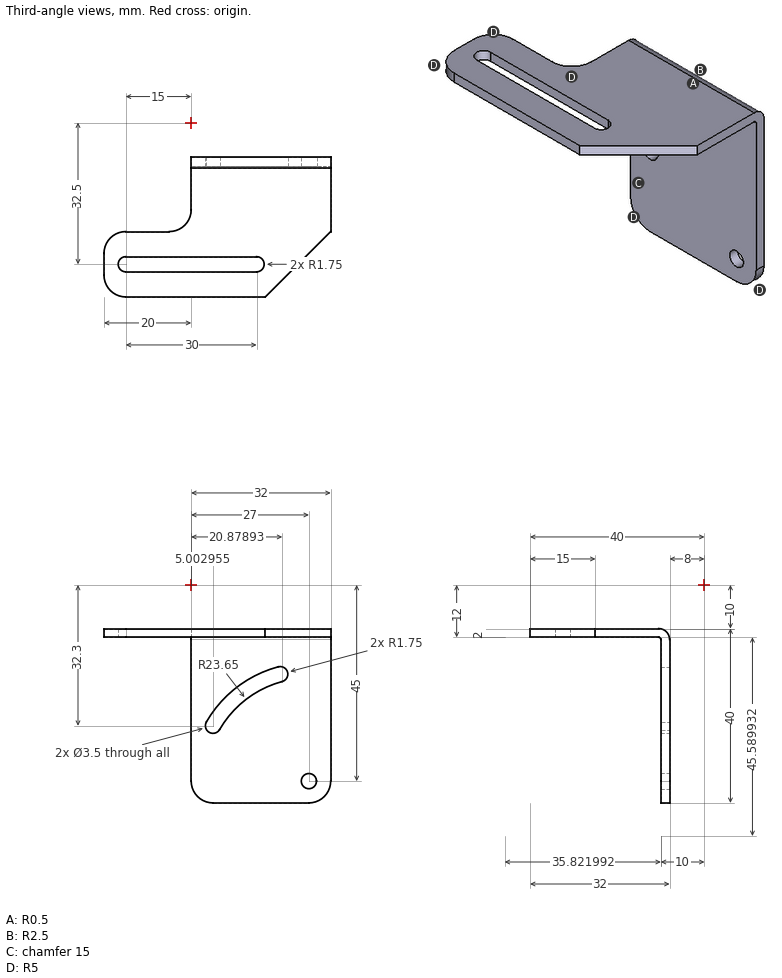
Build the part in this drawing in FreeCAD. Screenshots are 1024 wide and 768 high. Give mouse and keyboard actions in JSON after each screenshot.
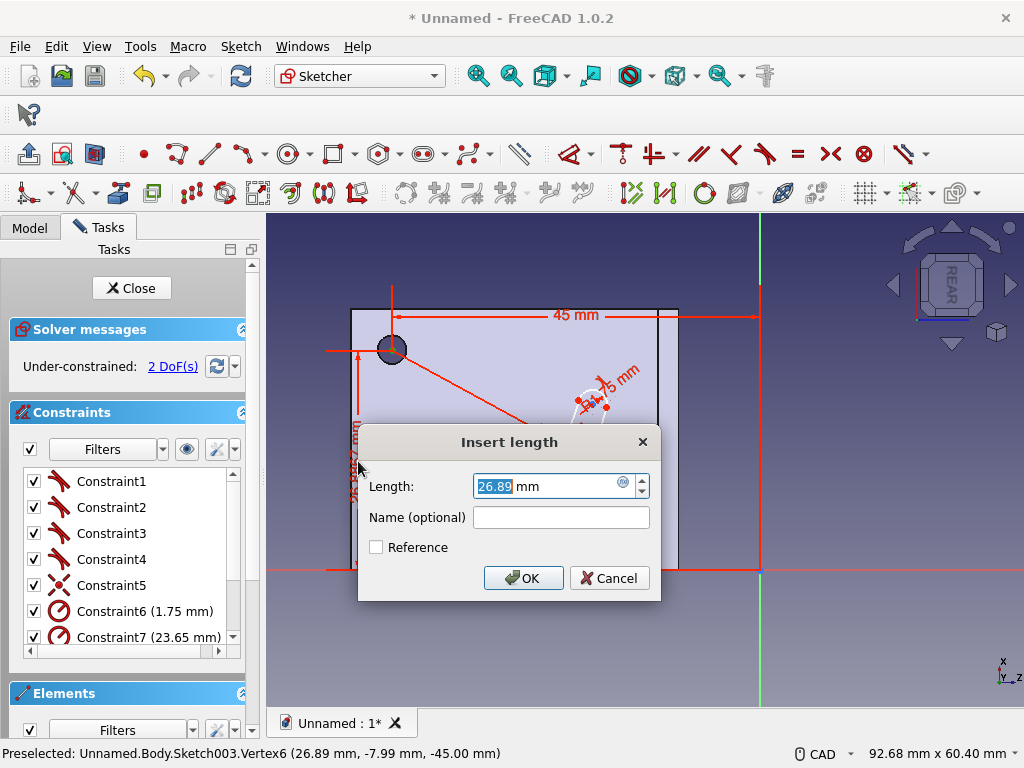
{"action": "type", "text": "27"}
{"action": "key", "text": "Return"}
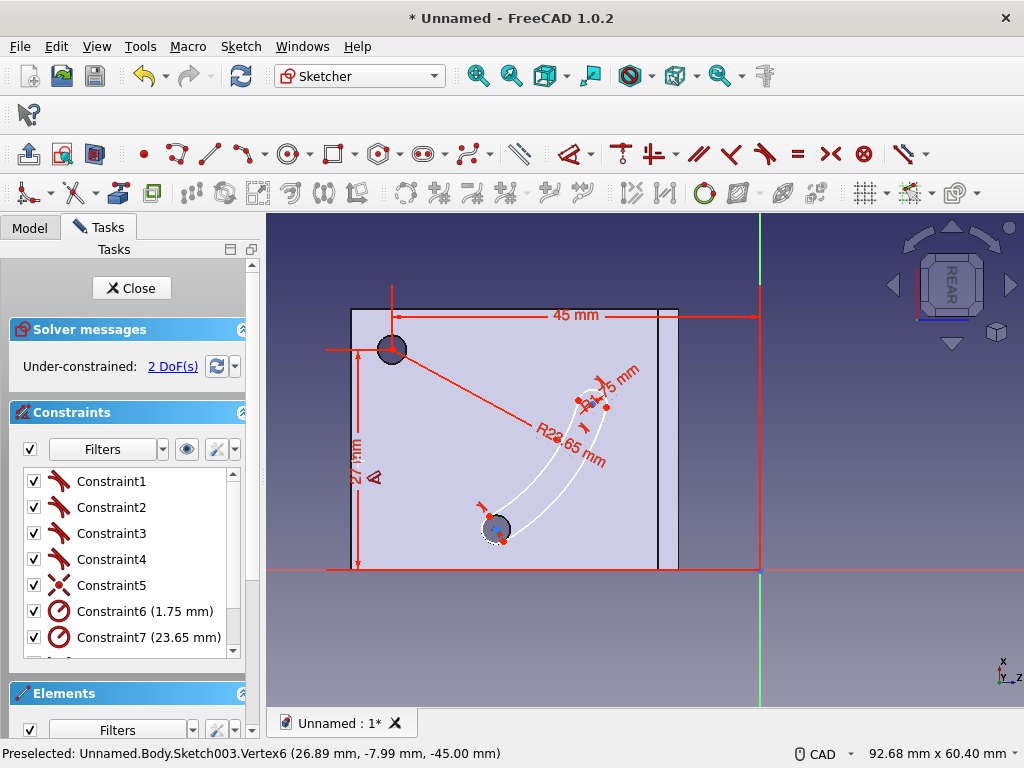
{"action": "left_click", "coordinate": [496, 529]}
{"action": "left_click", "coordinate": [628, 604]}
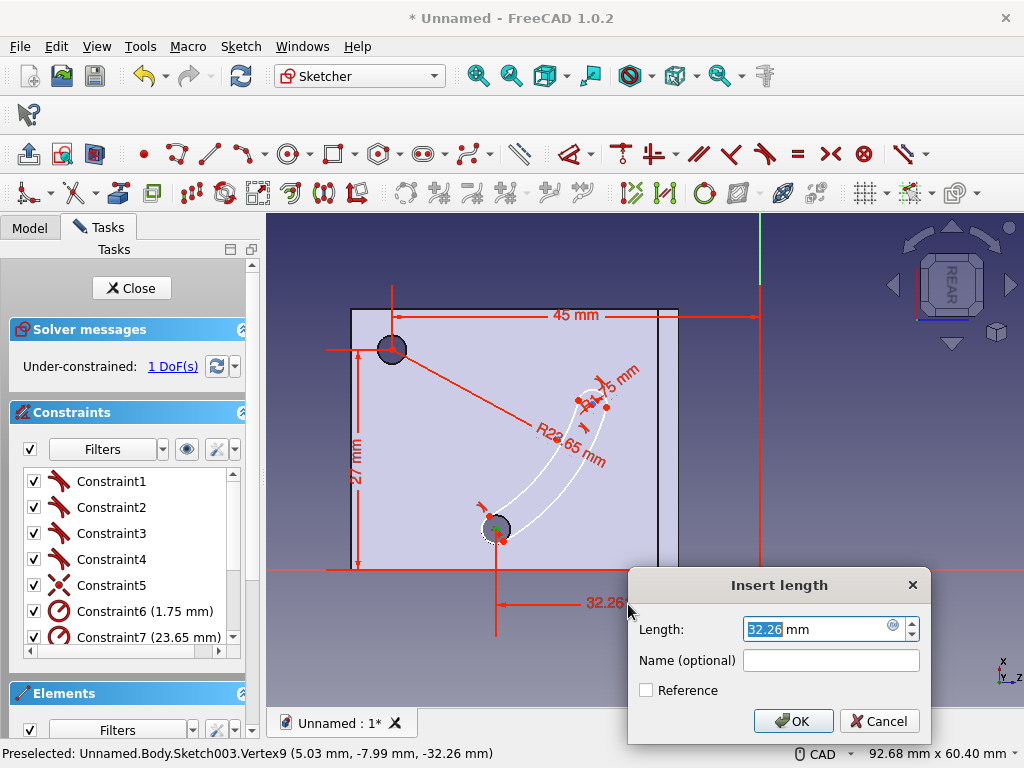
{"action": "type", "text": "32.3"}
{"action": "key", "text": "Return"}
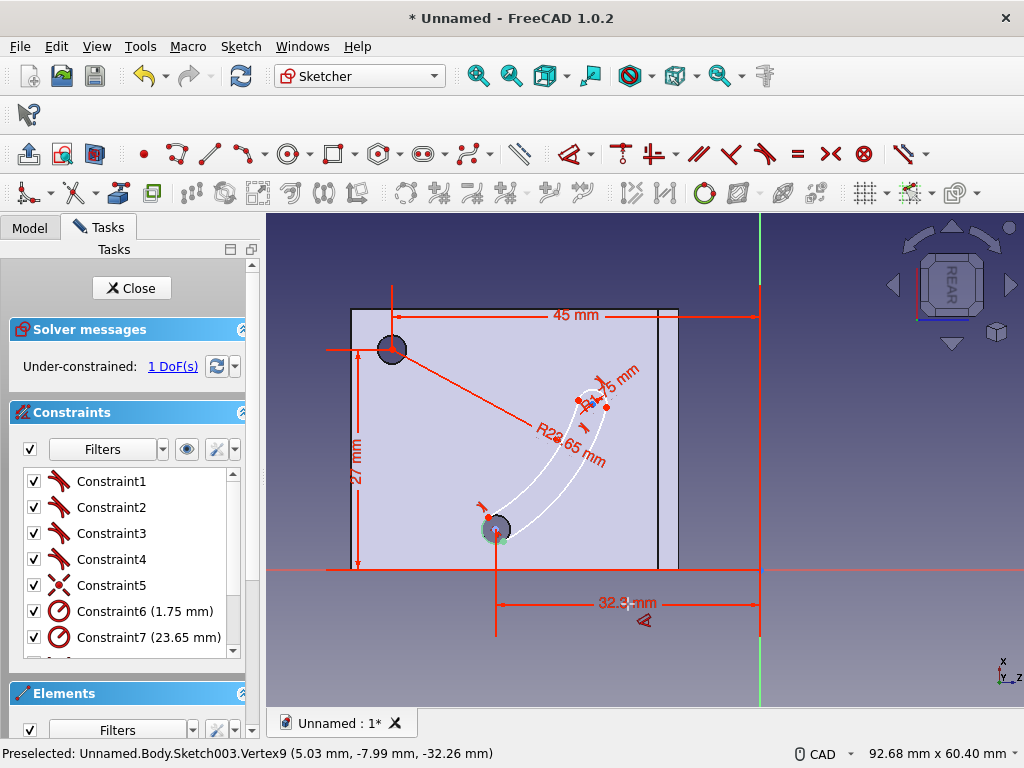
{"action": "left_click", "coordinate": [579, 400]}
{"action": "left_click", "coordinate": [794, 485]}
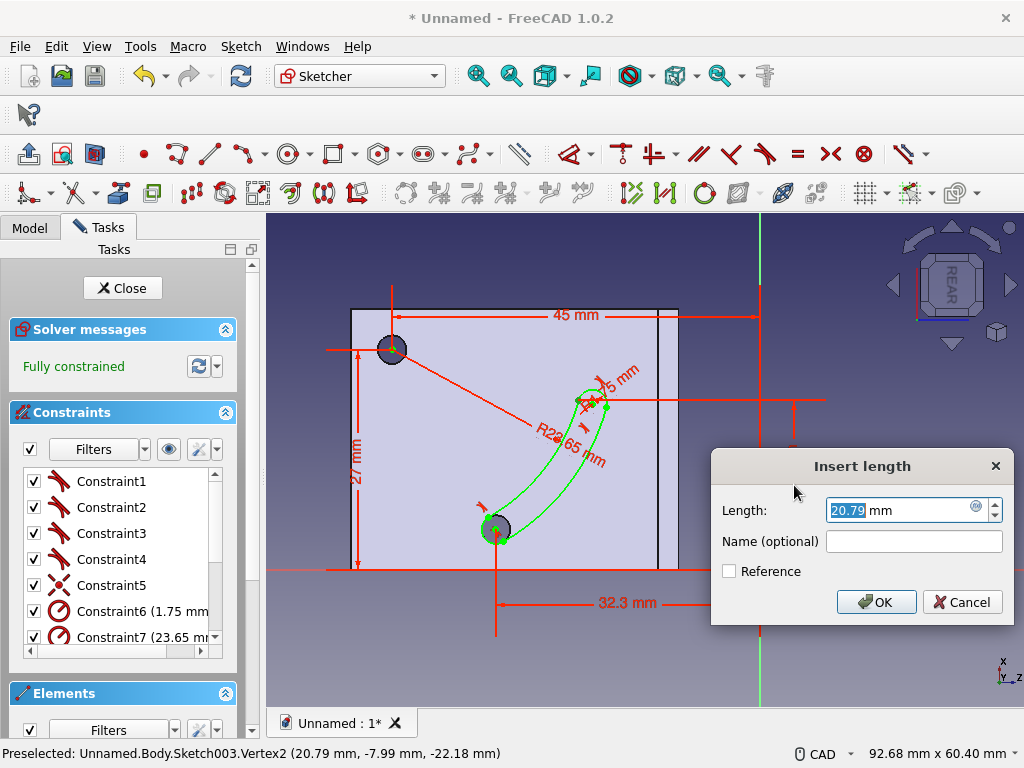
{"action": "type", "text": "20.87893"}
{"action": "key", "text": "Return"}
{"action": "key", "text": "Escape"}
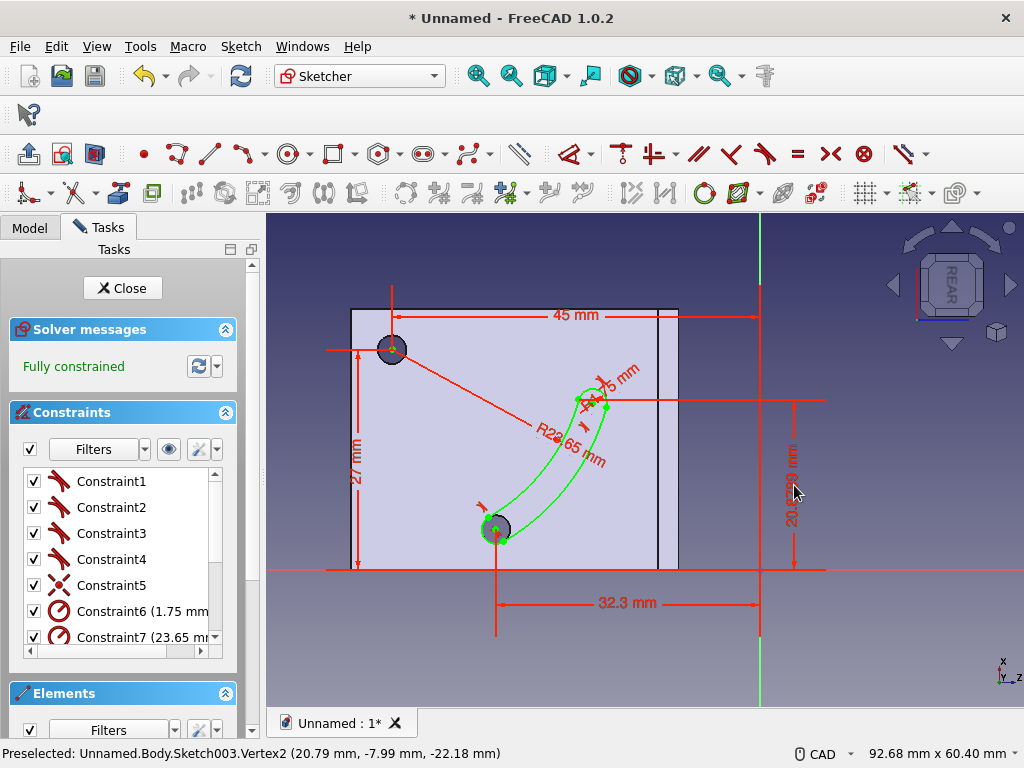
{"action": "left_click", "coordinate": [123, 288]}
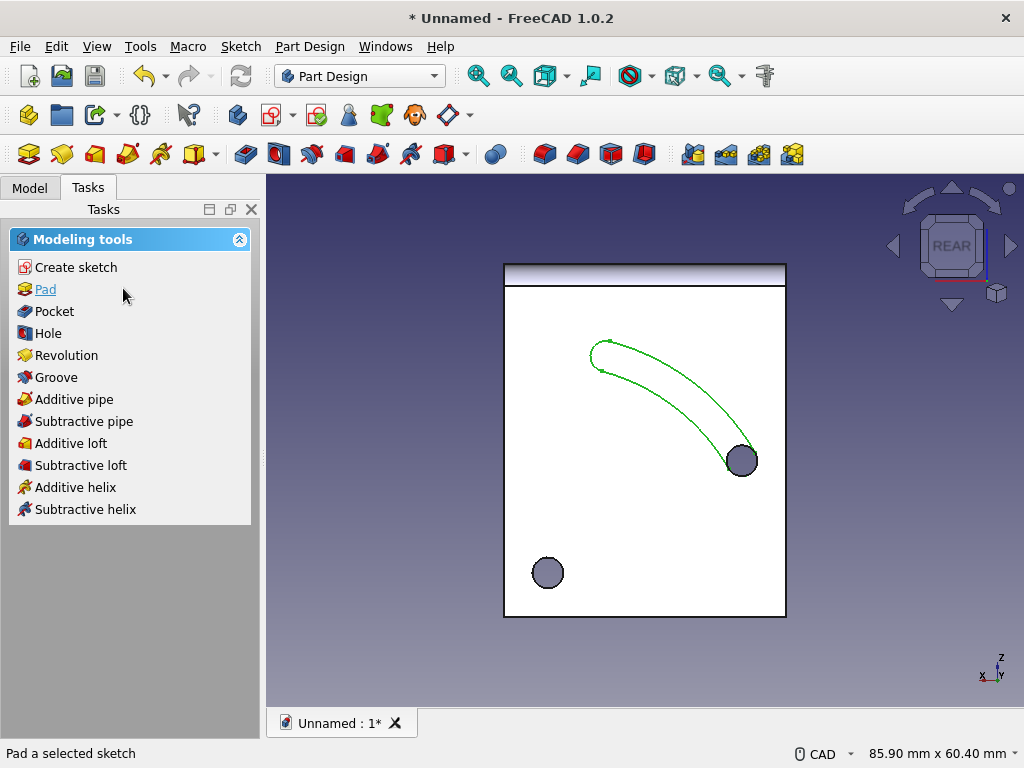
{"action": "left_click", "coordinate": [246, 154]}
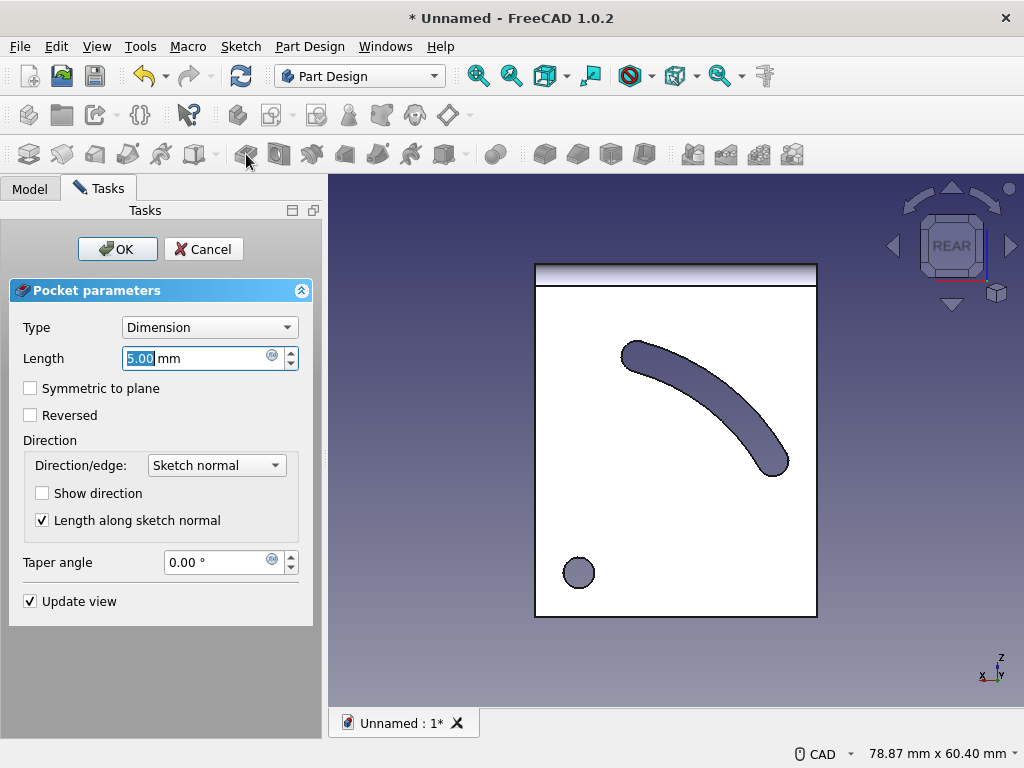
{"action": "left_click", "coordinate": [210, 328]}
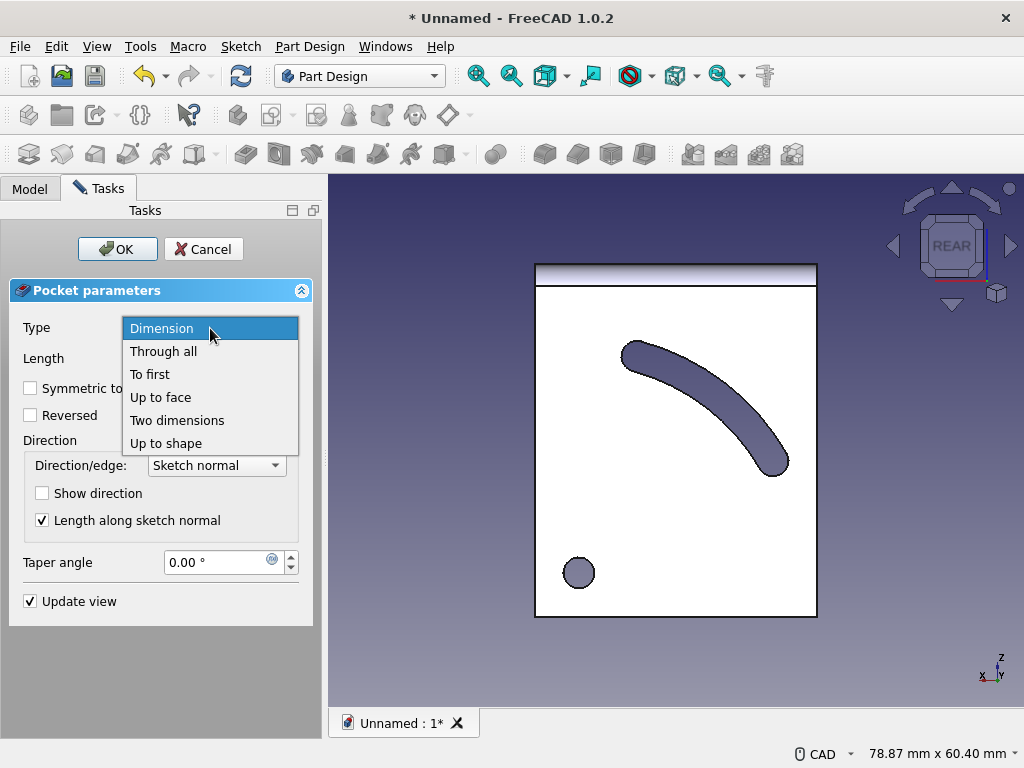
{"action": "left_click", "coordinate": [208, 374]}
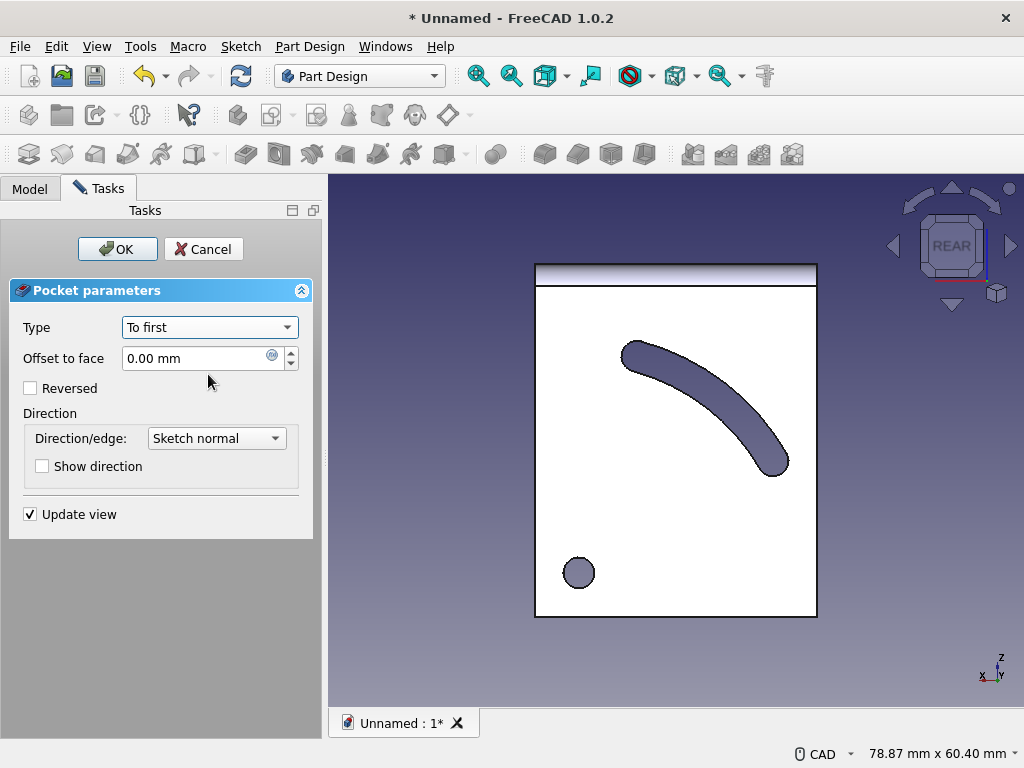
{"action": "left_click", "coordinate": [118, 249]}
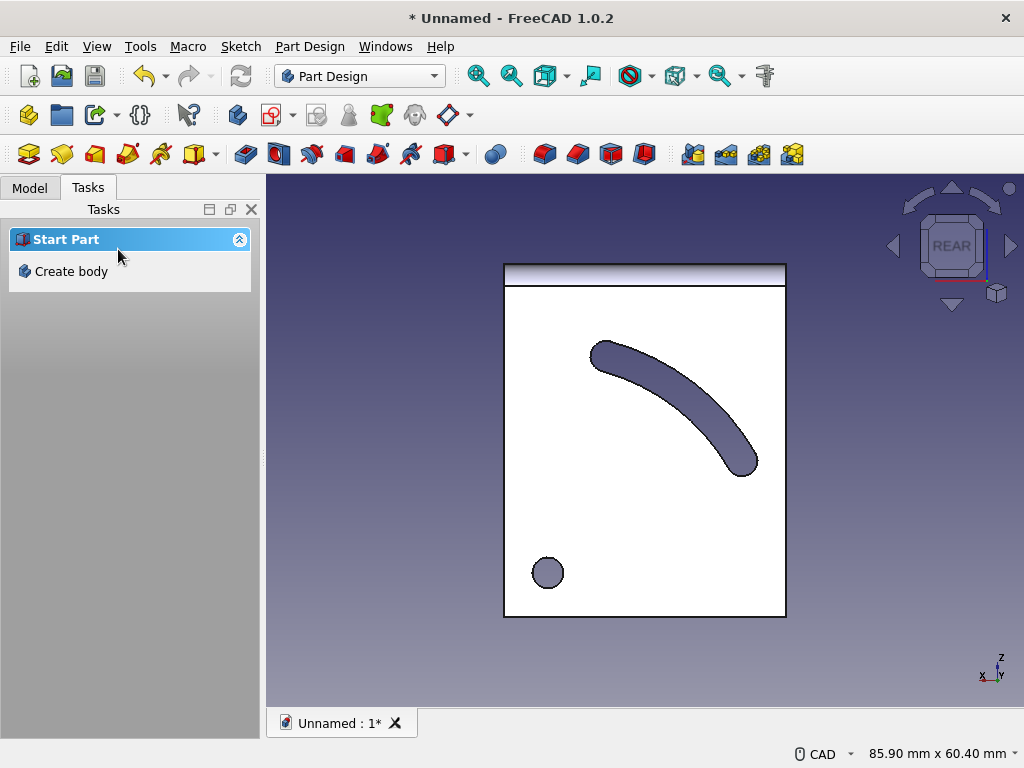
{"action": "key", "text": "6"}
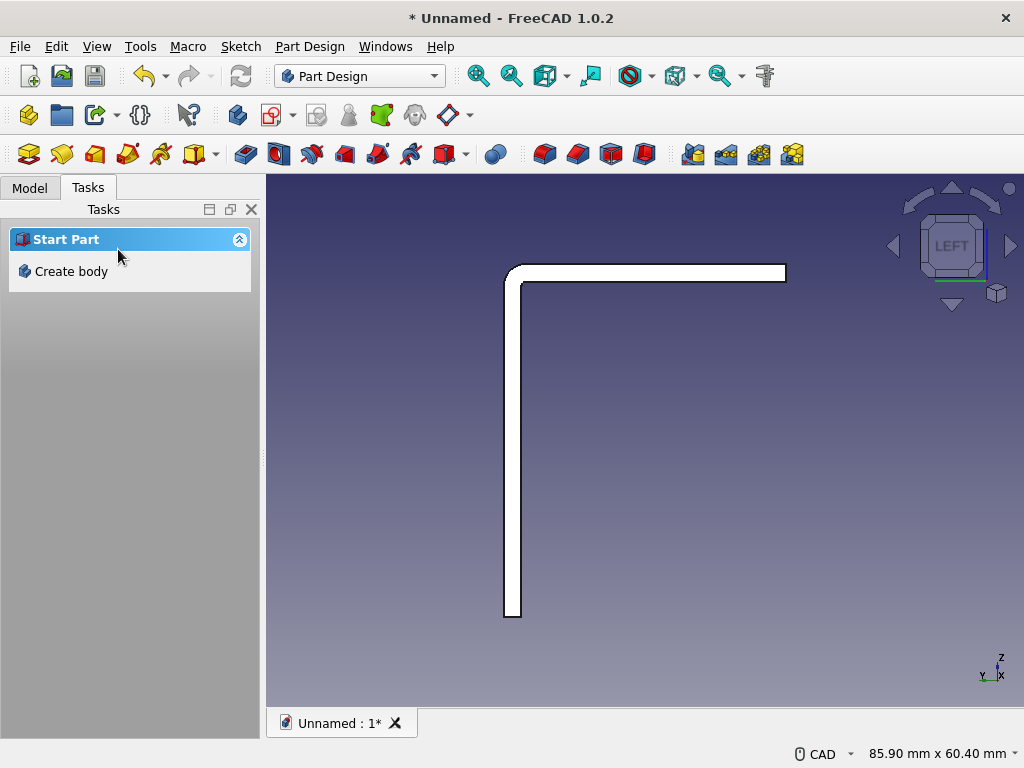
{"action": "left_click", "coordinate": [515, 273]}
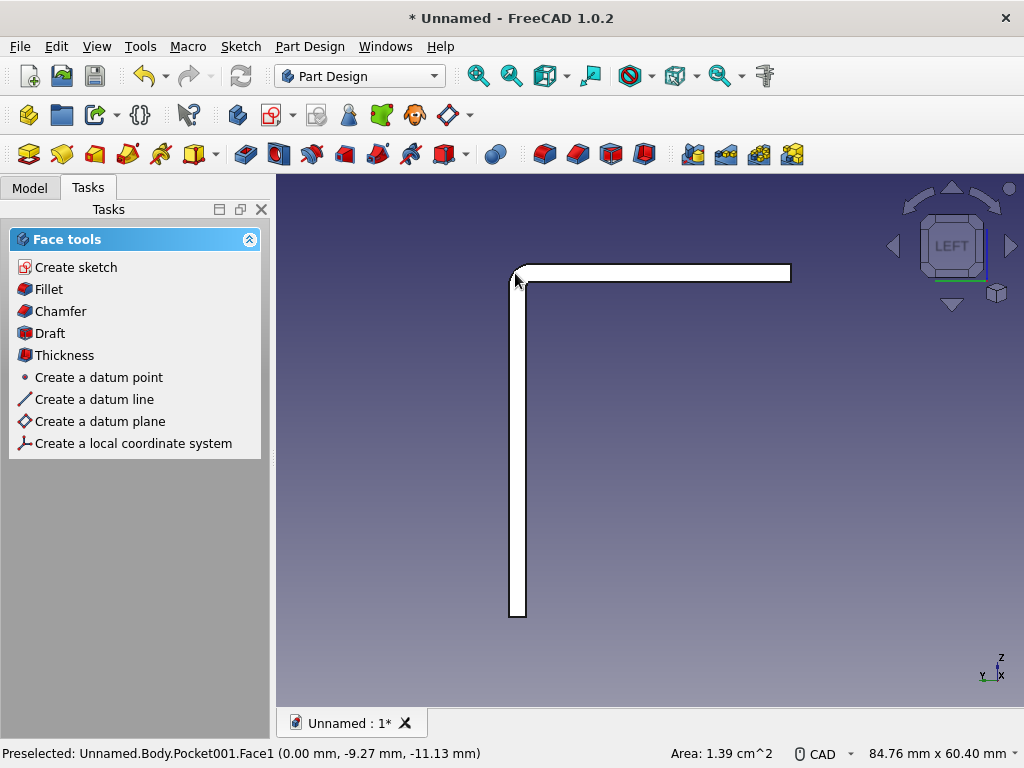
{"action": "left_click", "coordinate": [270, 116]}